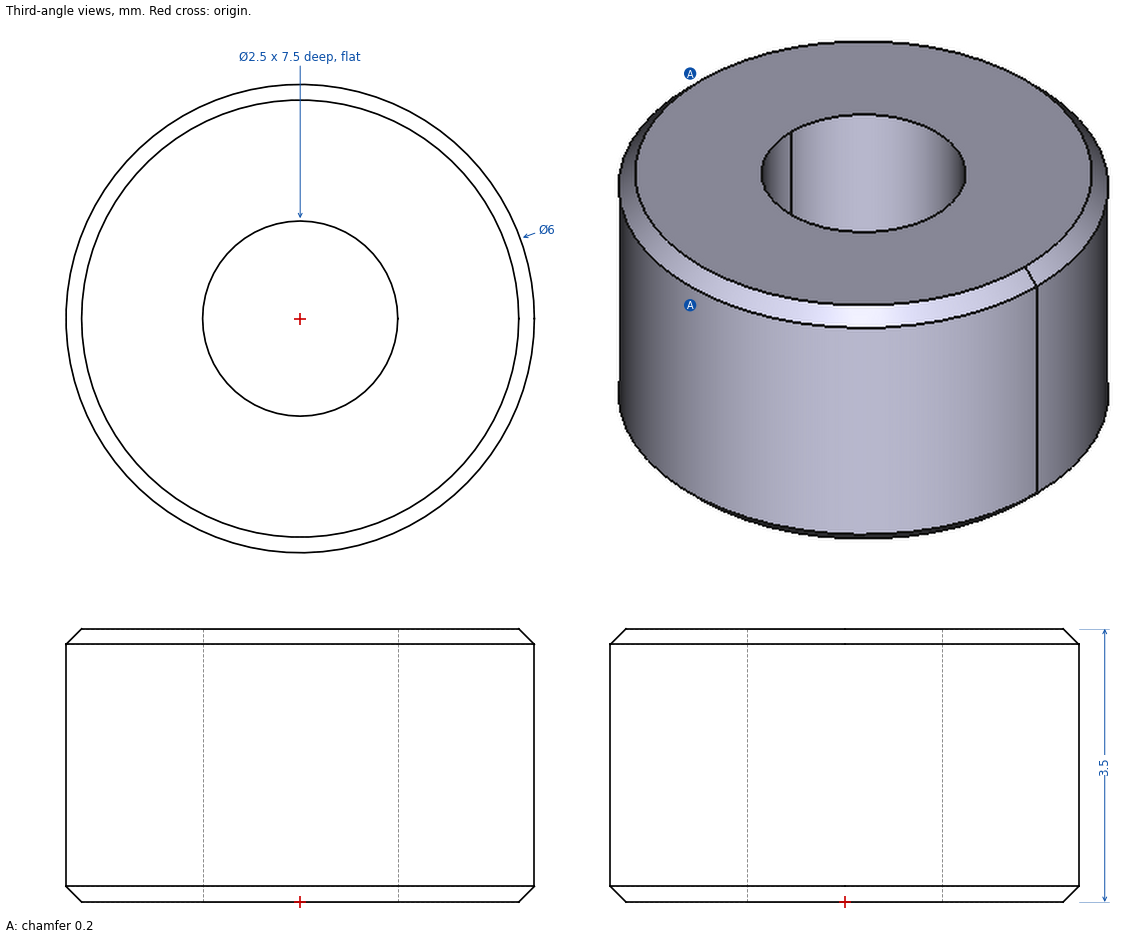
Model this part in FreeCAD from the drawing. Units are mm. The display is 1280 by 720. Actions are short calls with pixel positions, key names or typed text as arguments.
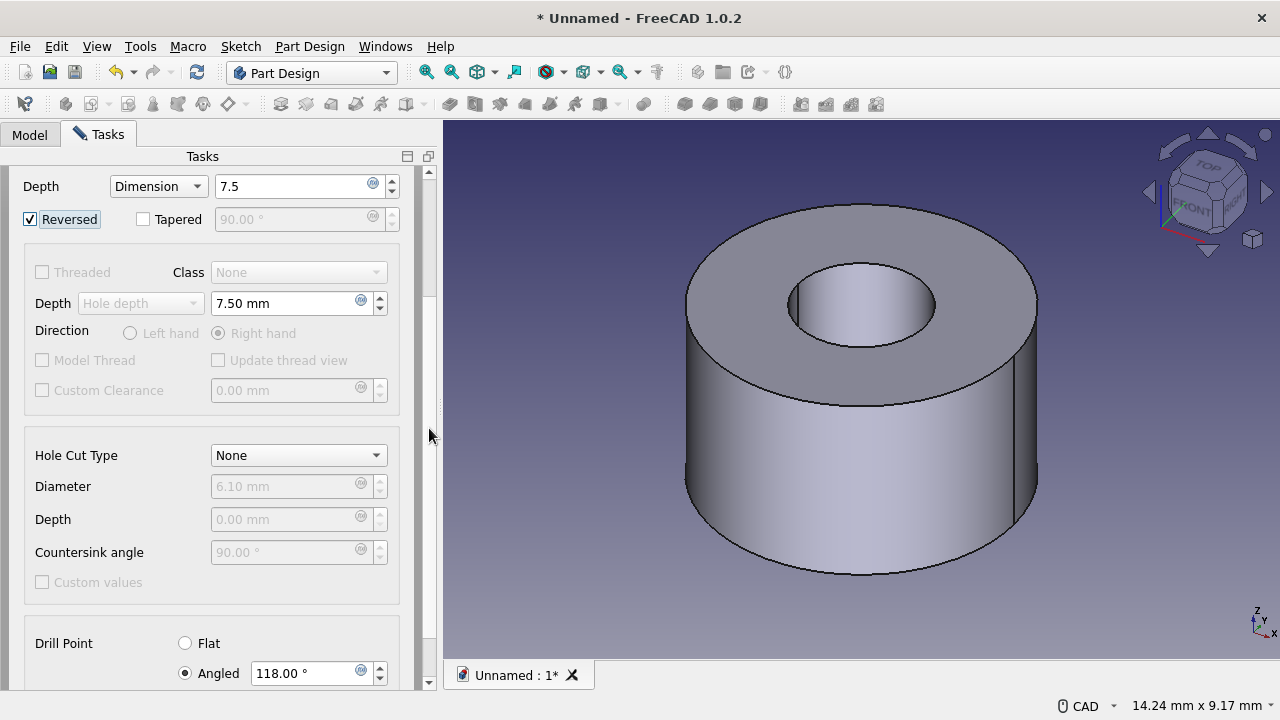
click(186, 583)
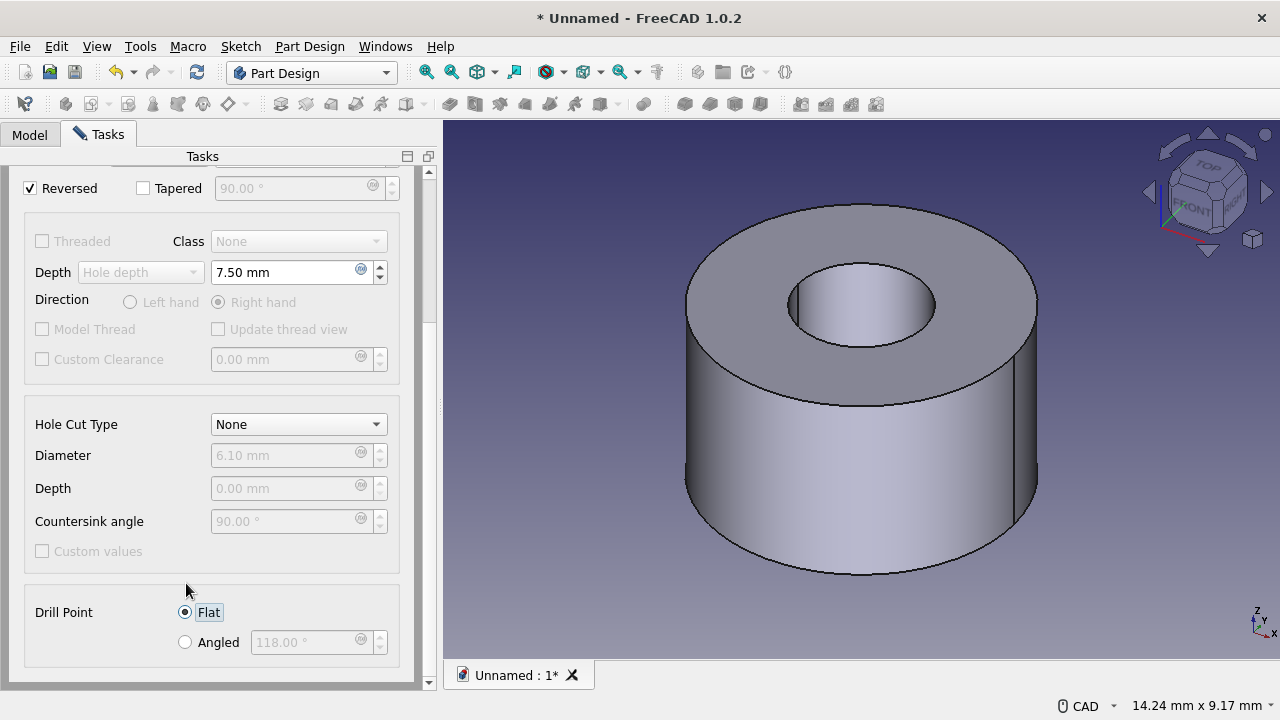
scroll(429, 428, up, 5)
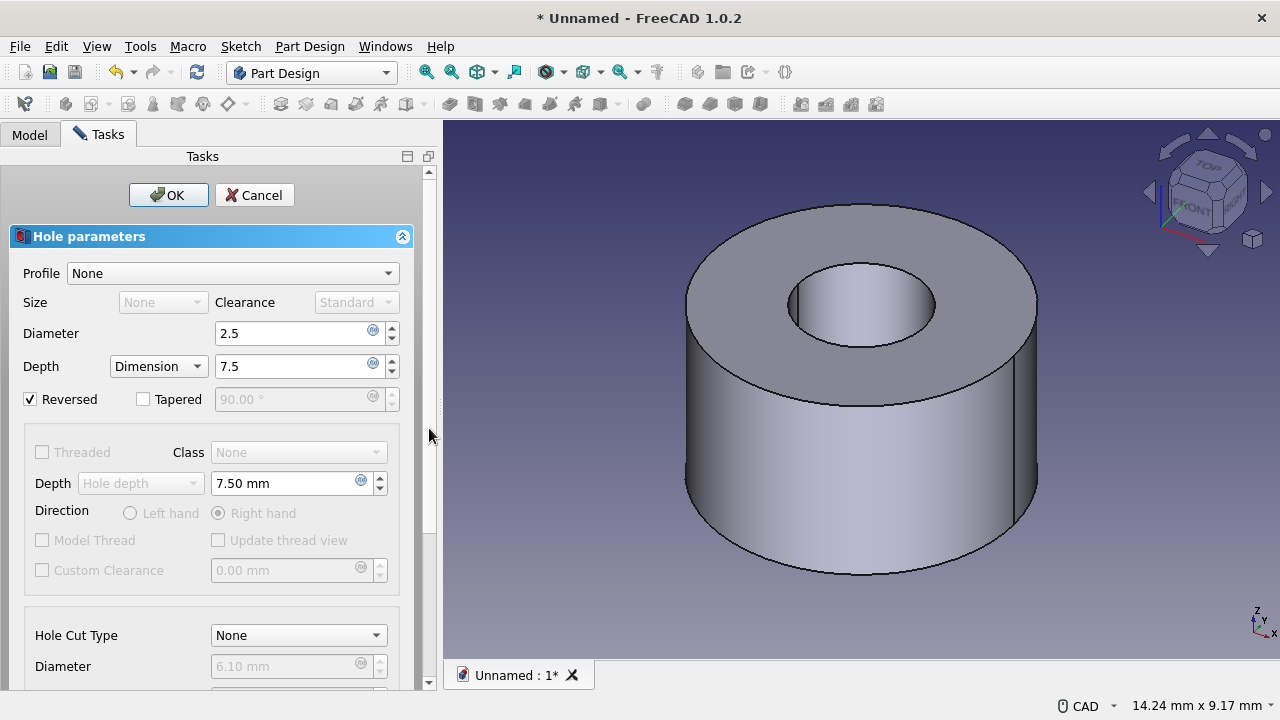
click(169, 195)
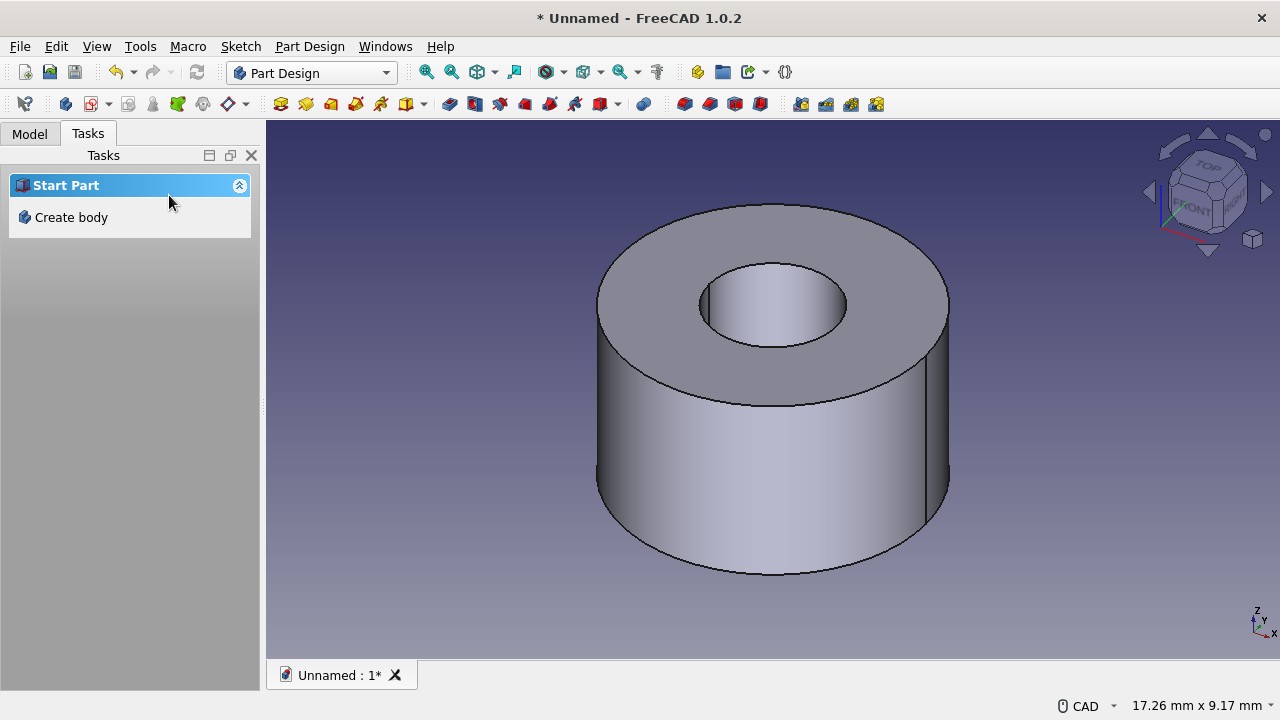
click(598, 315)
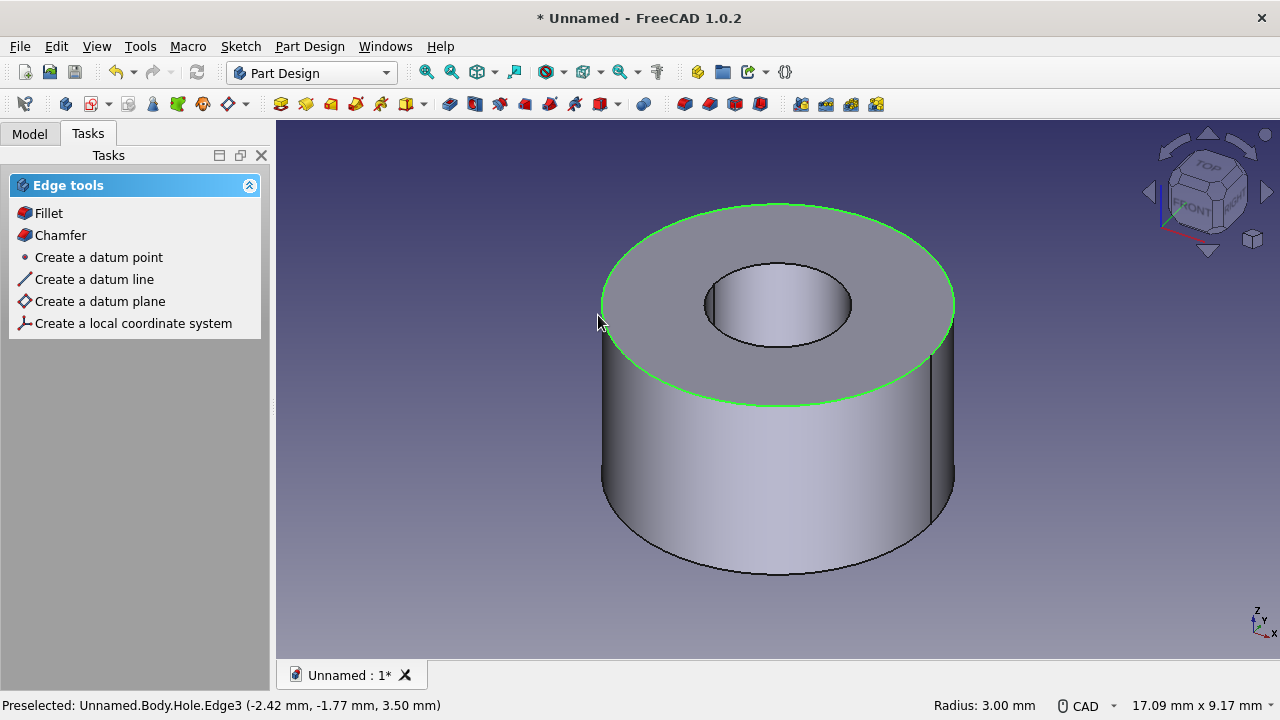
key(0)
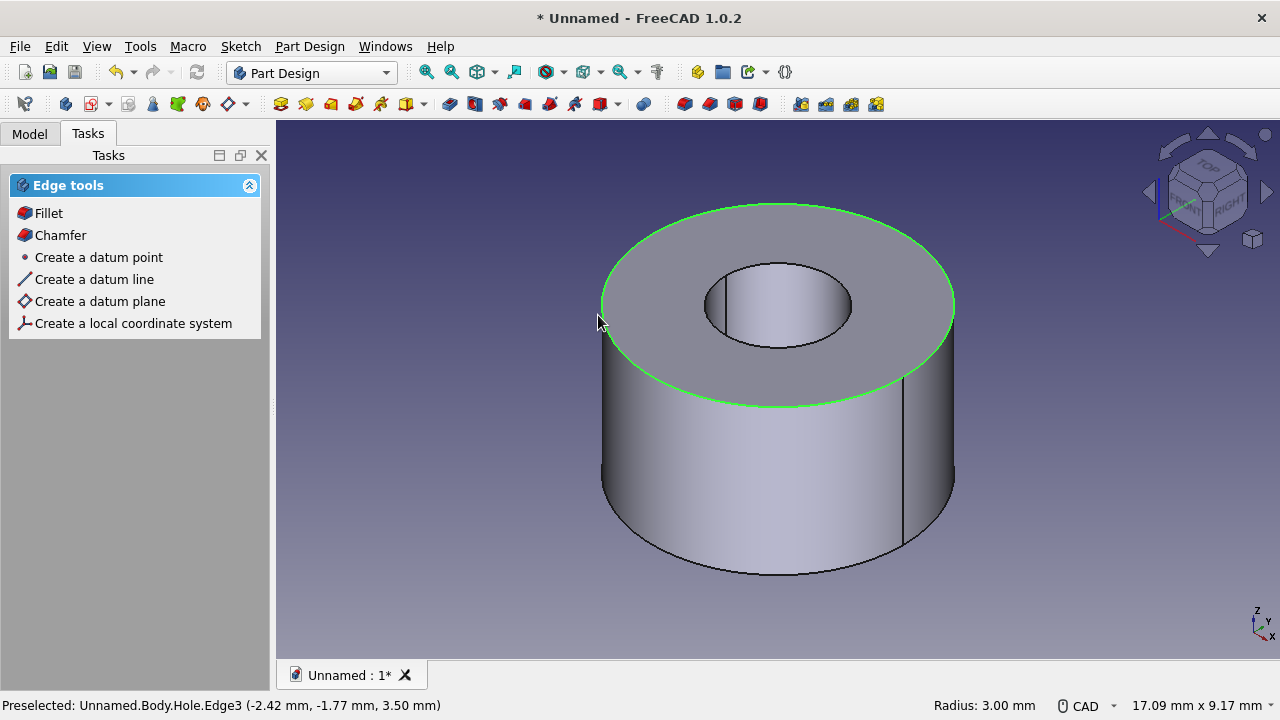
click(621, 519, ctrl)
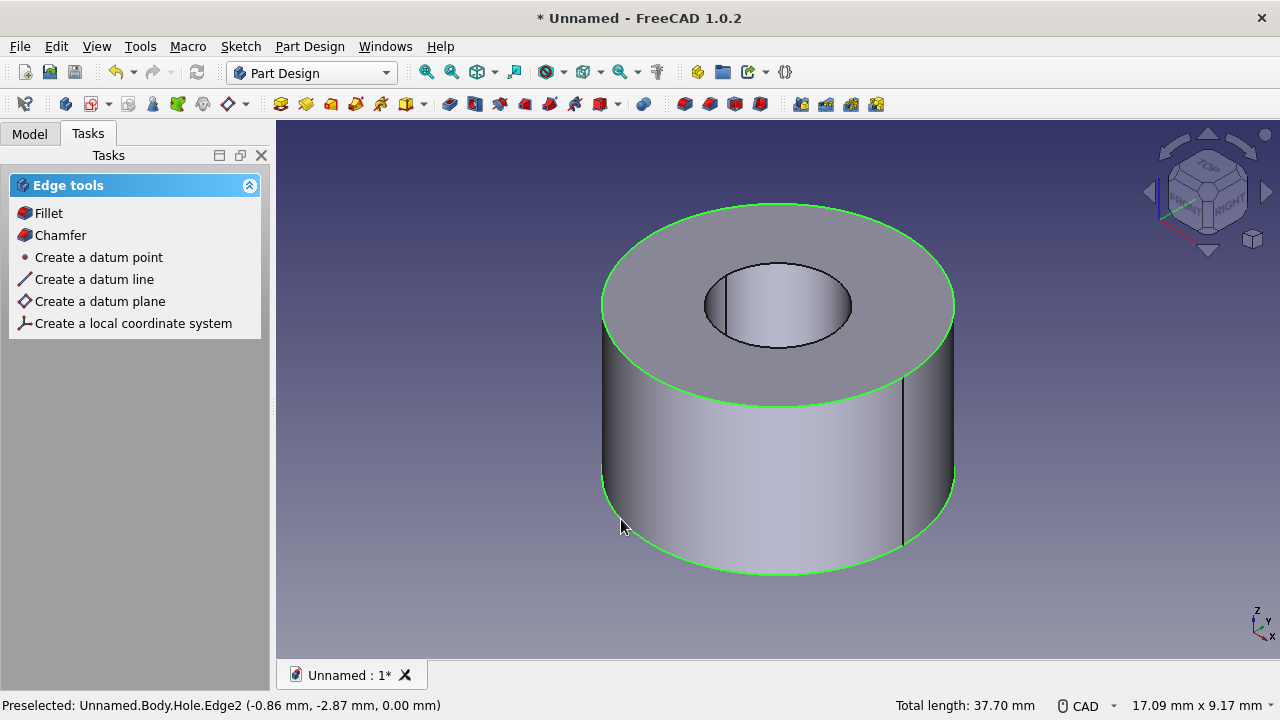
click(710, 104)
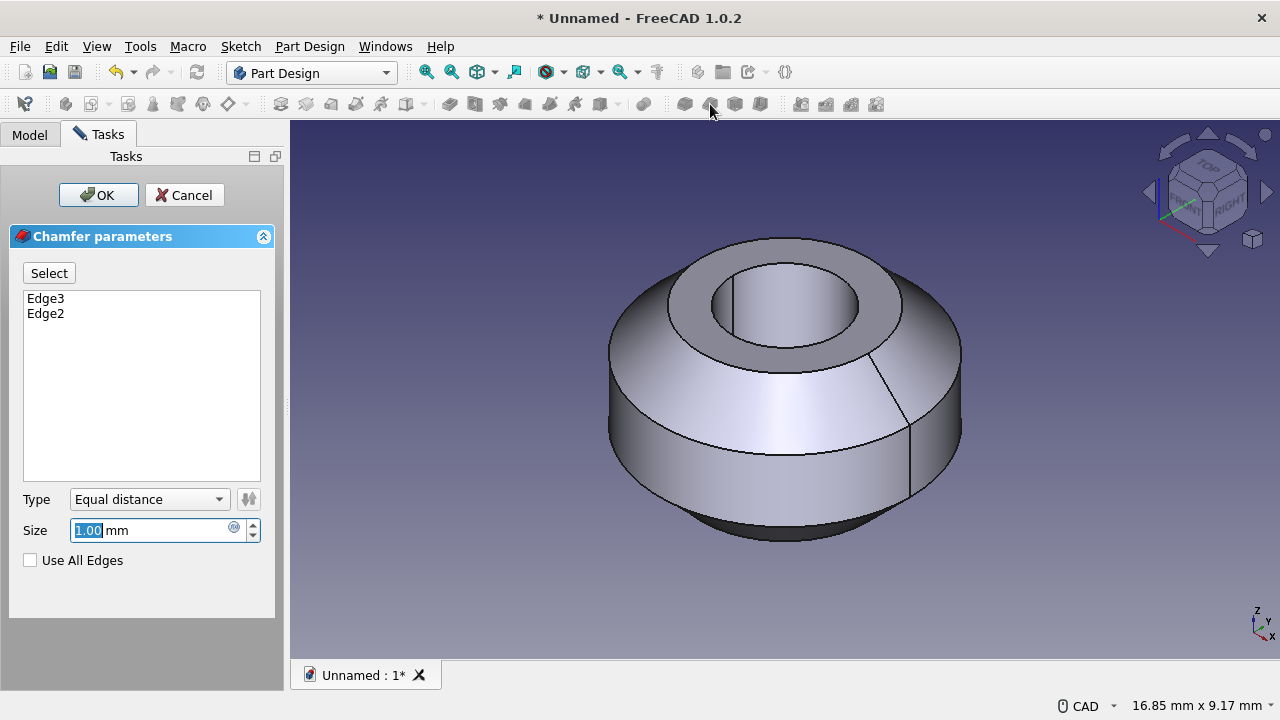
text(0.2)
key(Tab)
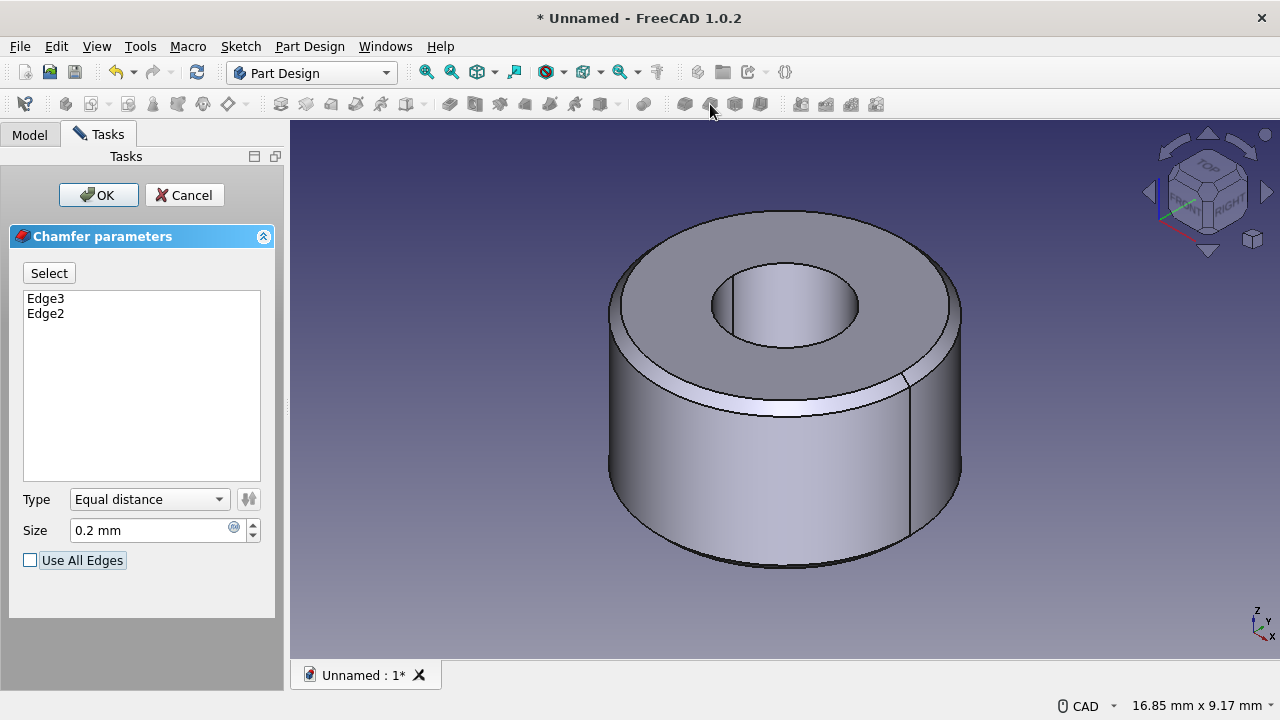
click(99, 195)